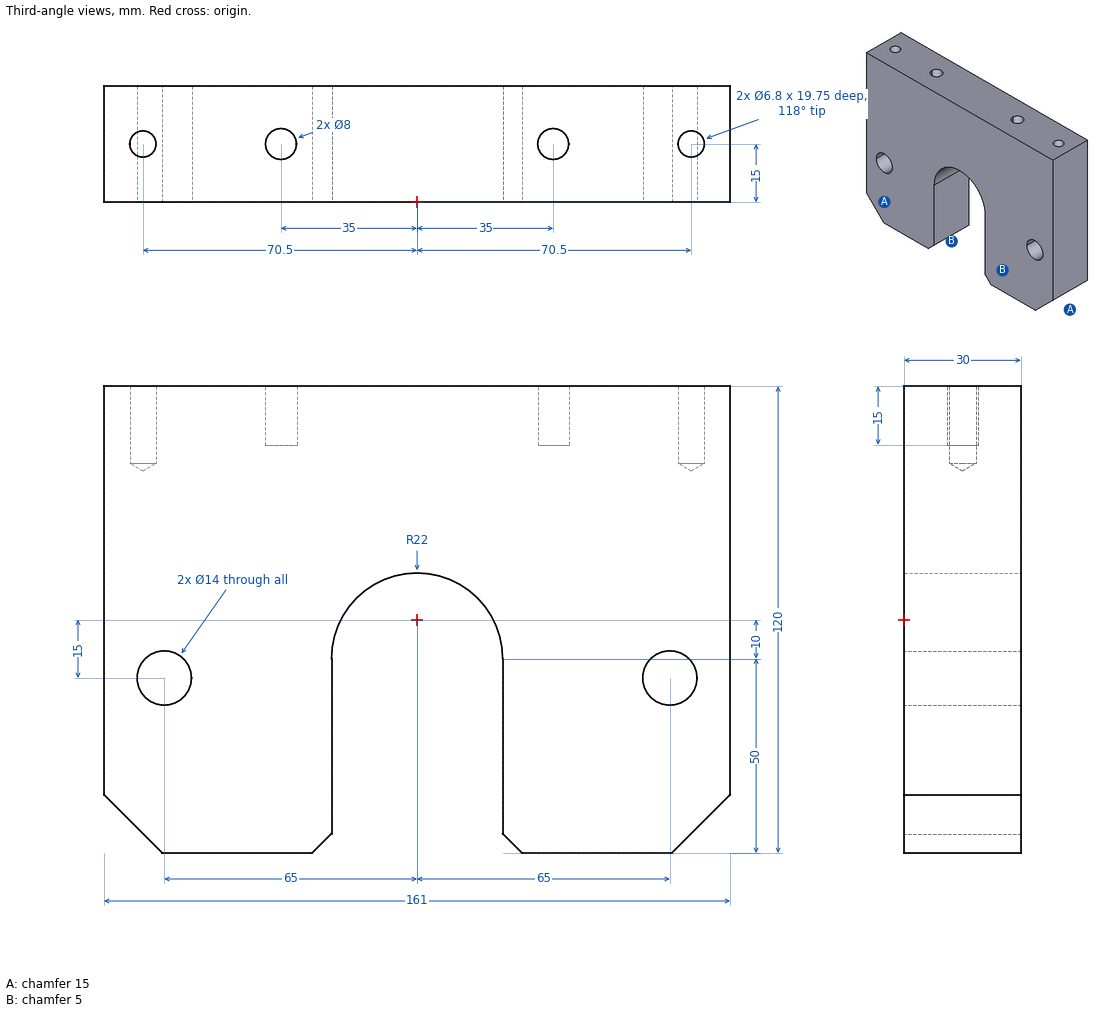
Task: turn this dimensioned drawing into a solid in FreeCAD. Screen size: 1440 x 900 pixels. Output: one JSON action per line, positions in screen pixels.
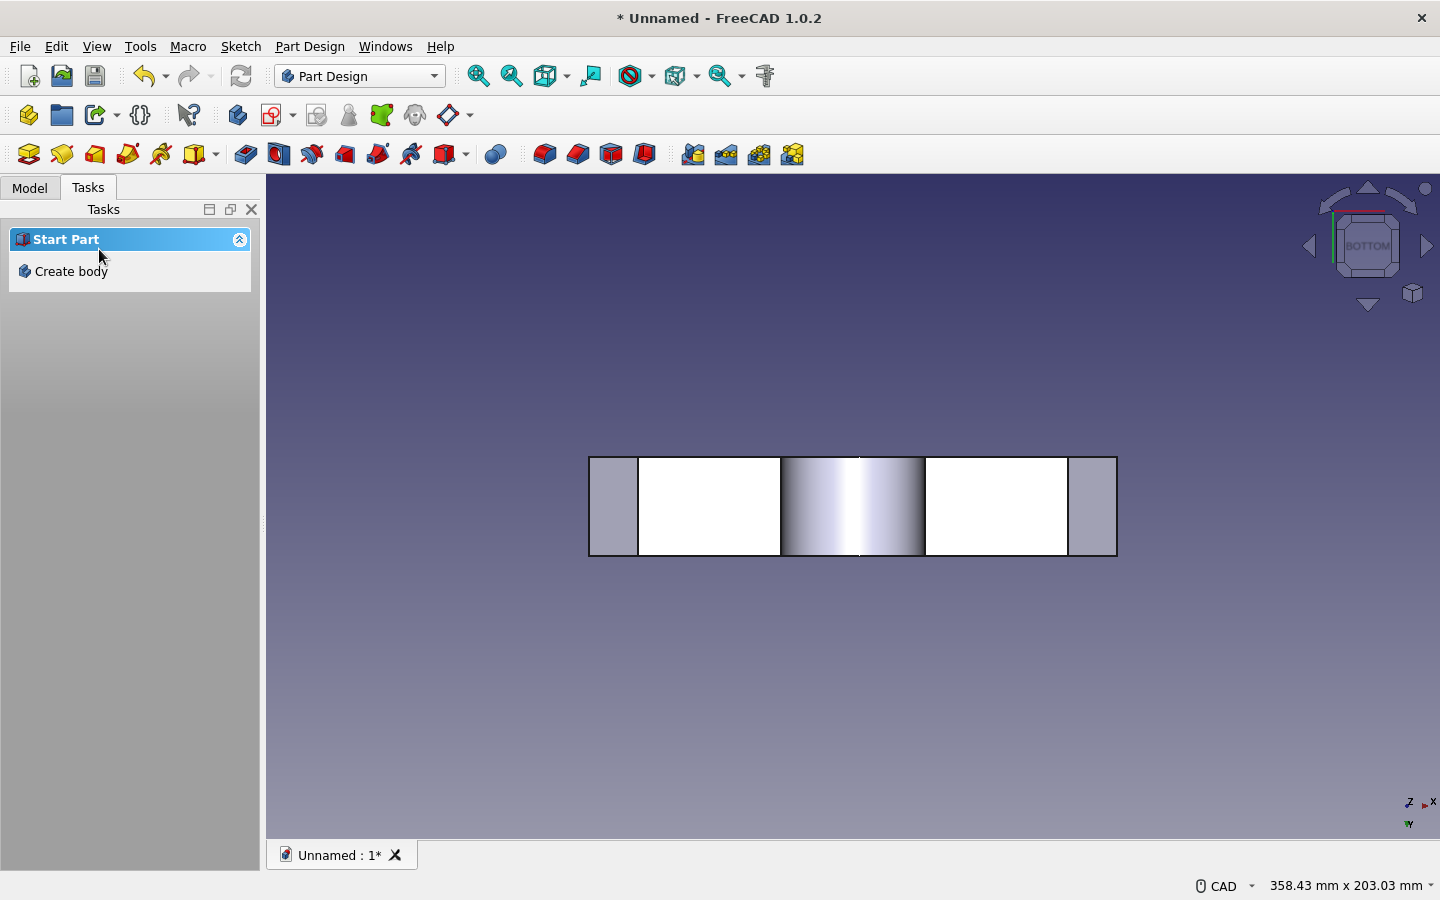
{"action": "key", "text": "v f"}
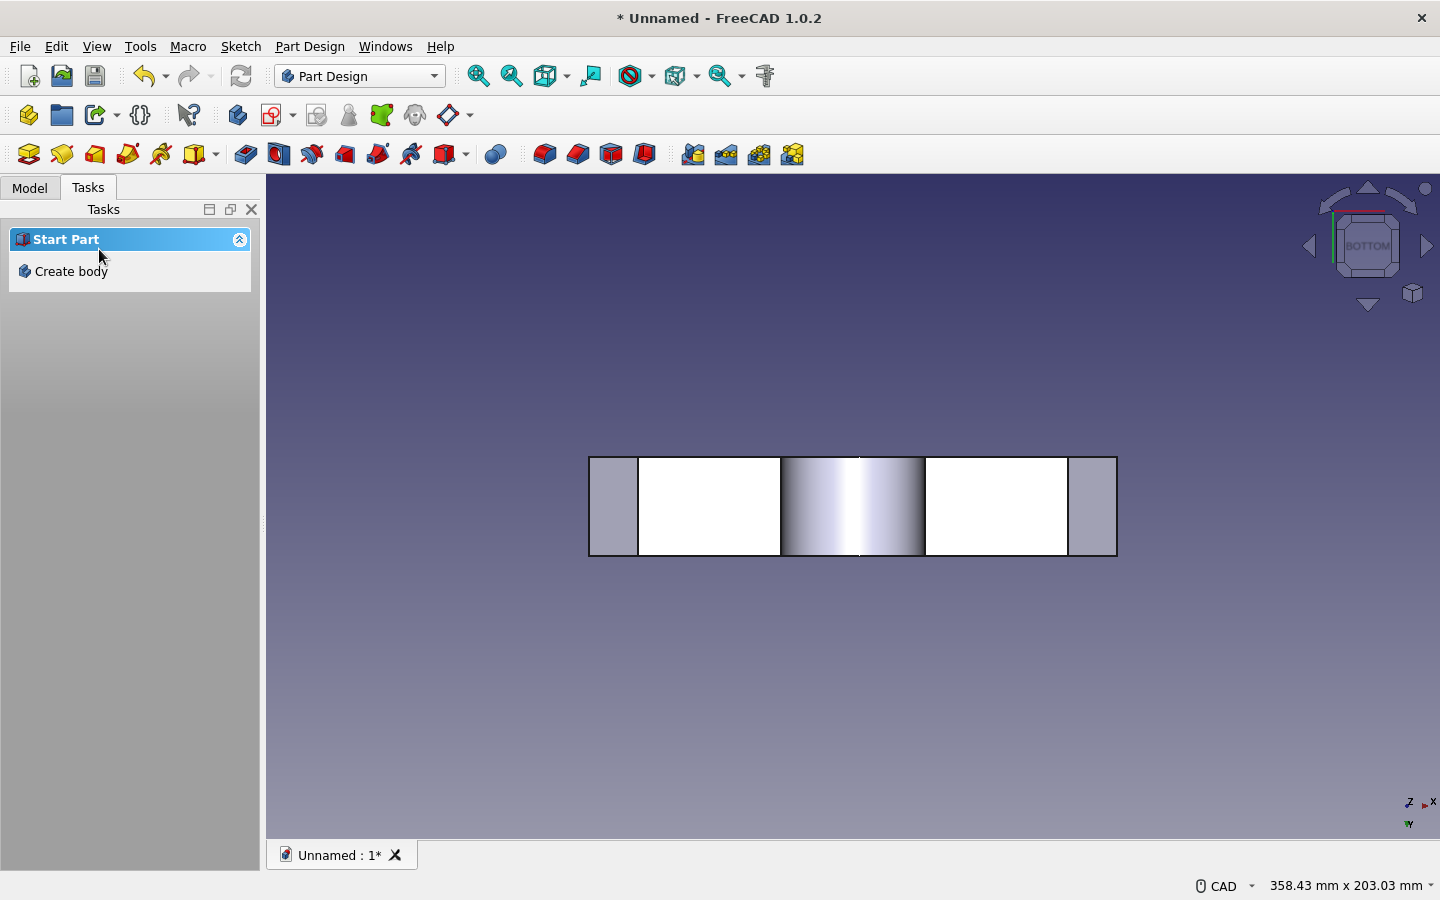
{"action": "left_click", "coordinate": [781, 505]}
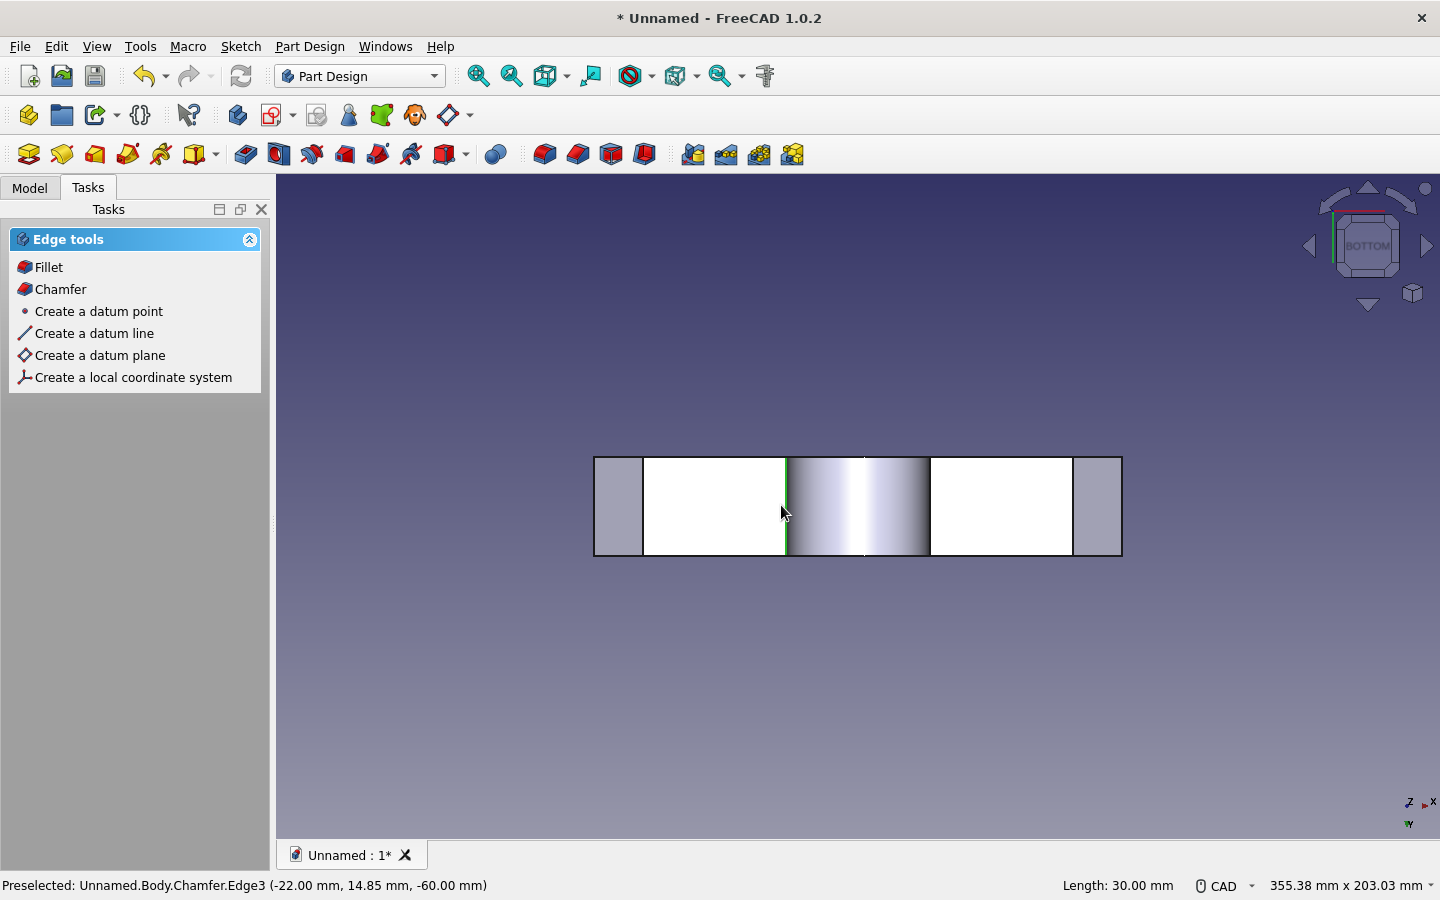
{"action": "left_click", "coordinate": [930, 505], "text": "ctrl"}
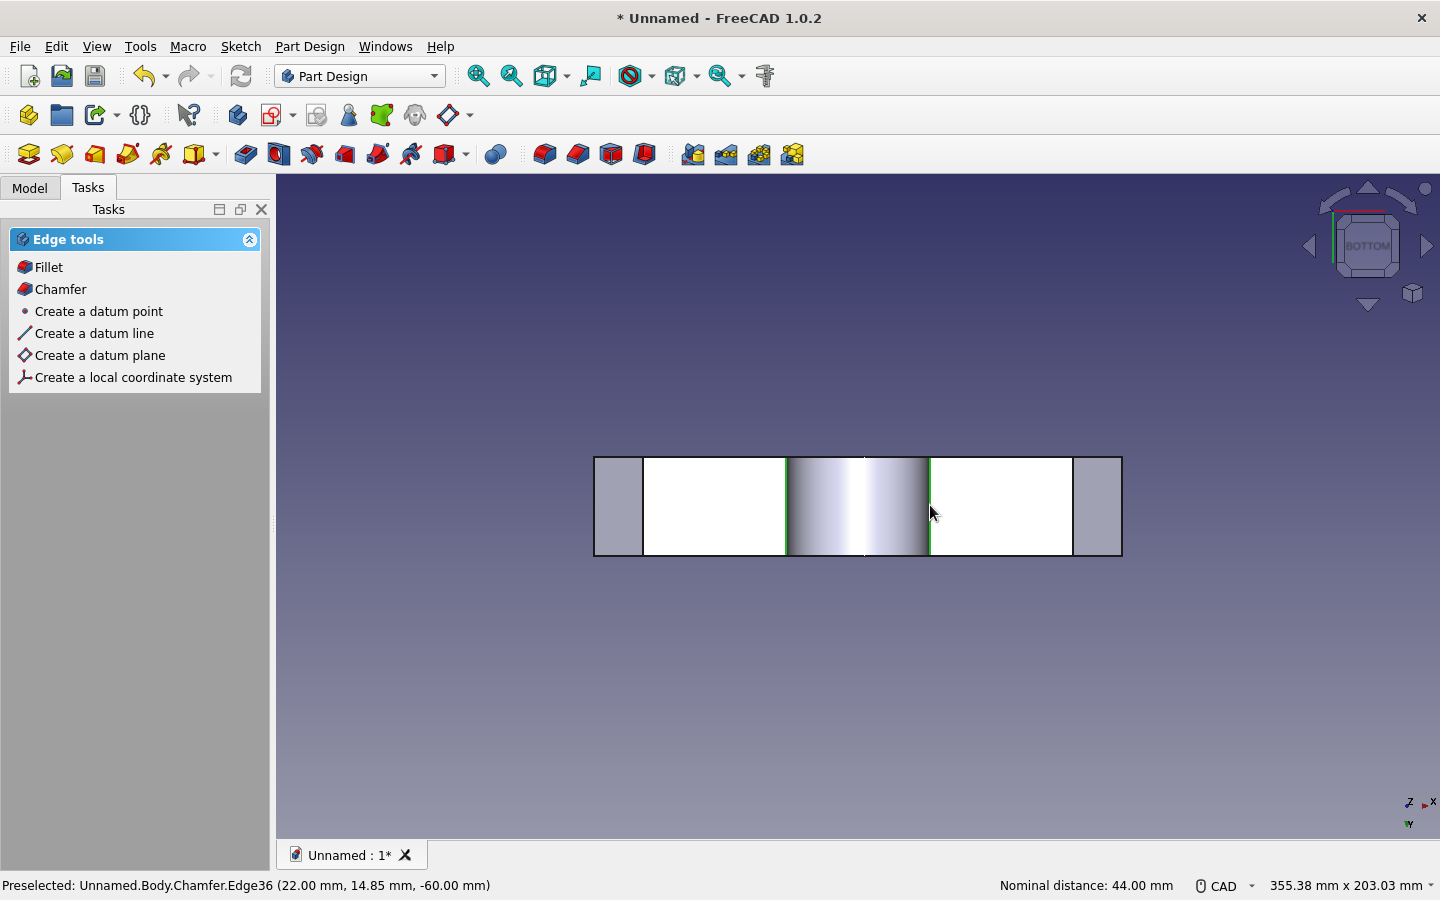
{"action": "left_click", "coordinate": [578, 154]}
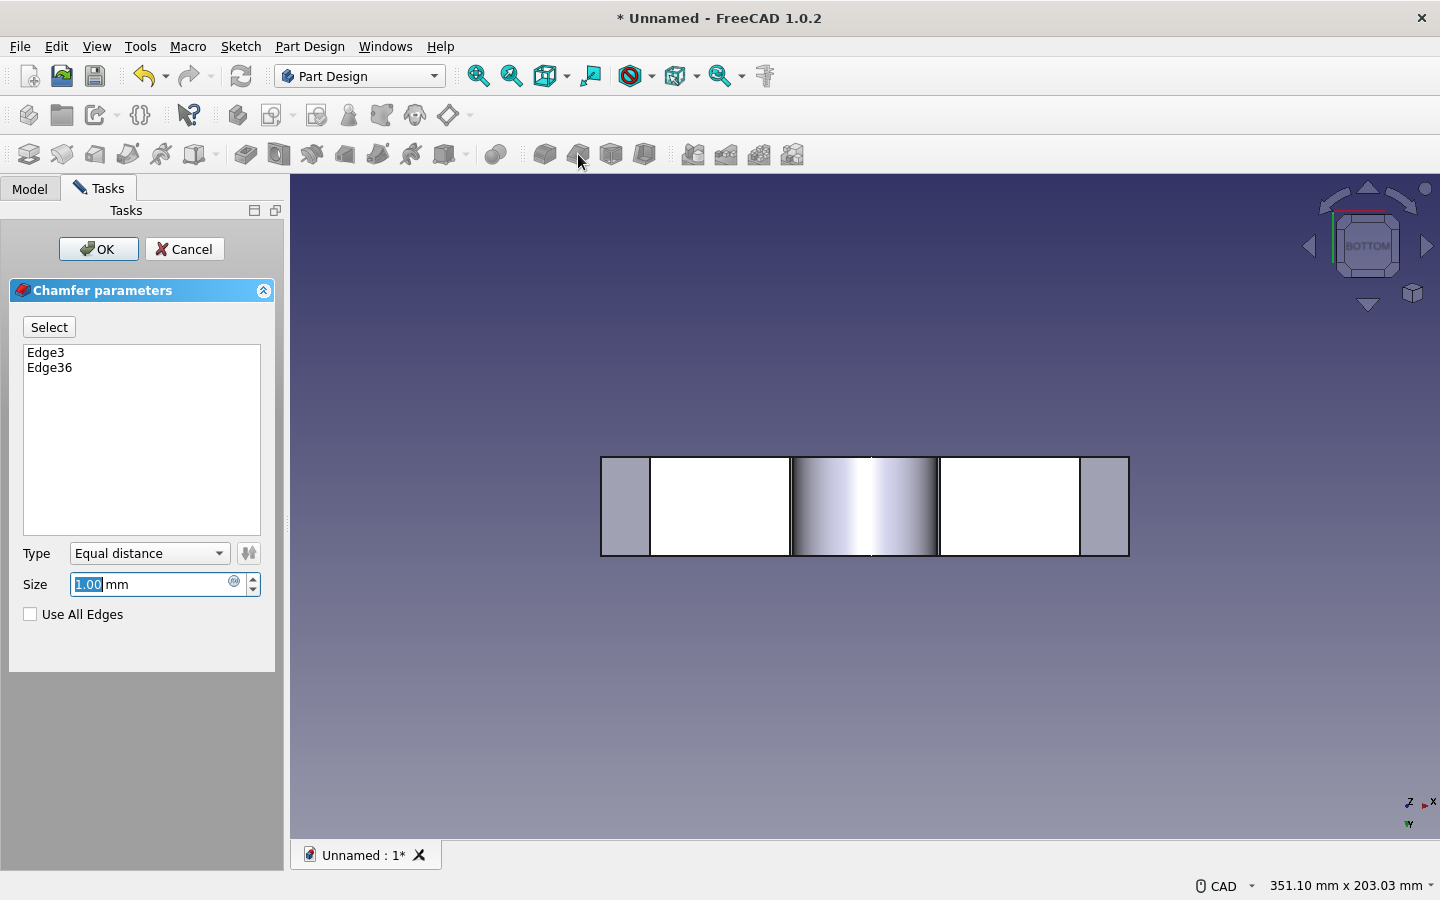
{"action": "type", "text": "5"}
{"action": "key", "text": "Tab"}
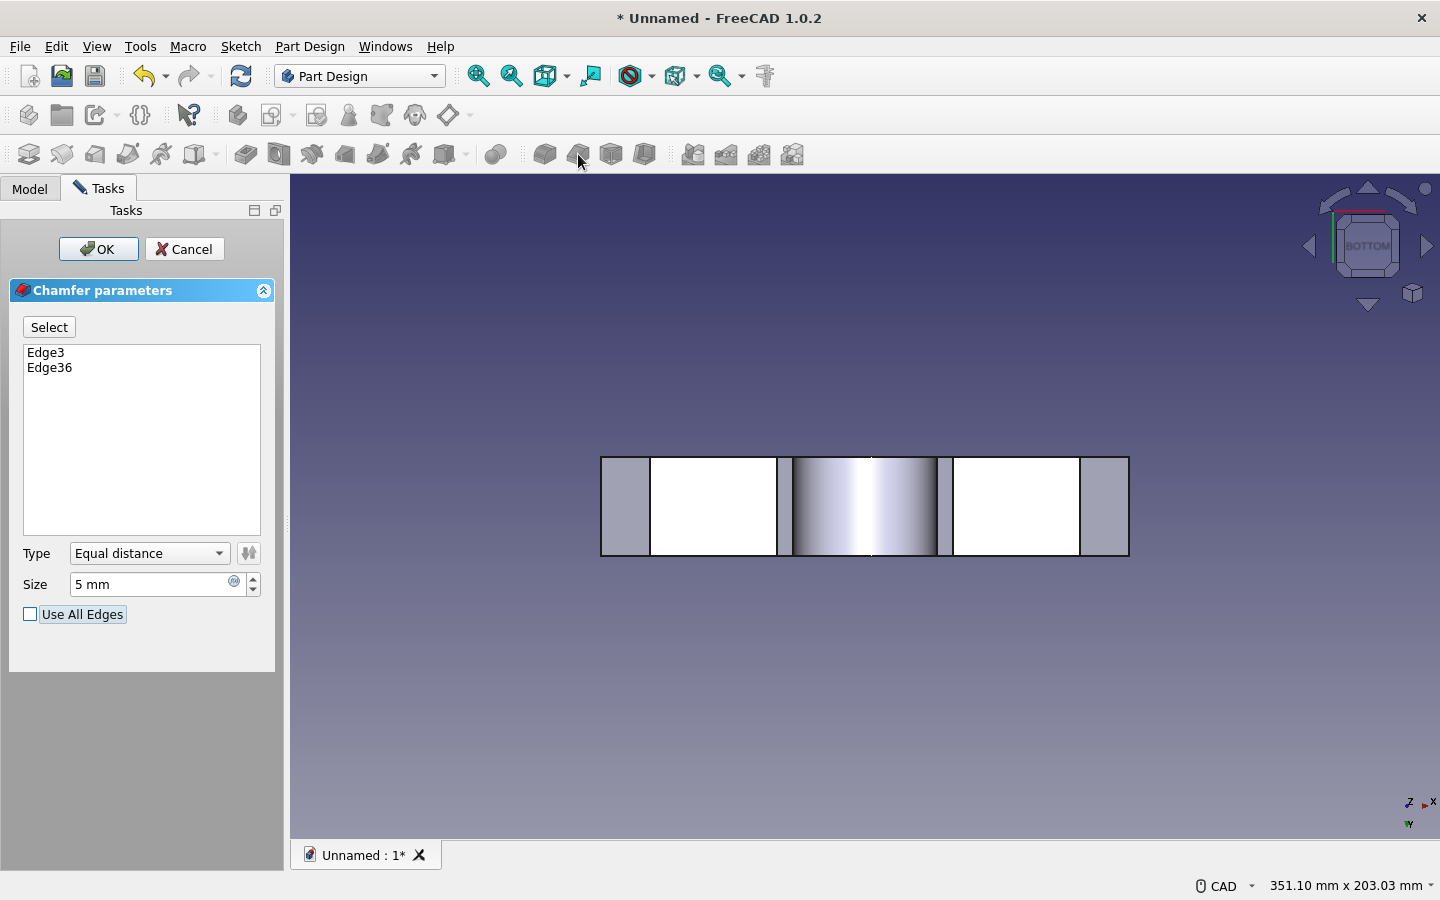
{"action": "left_click", "coordinate": [99, 249]}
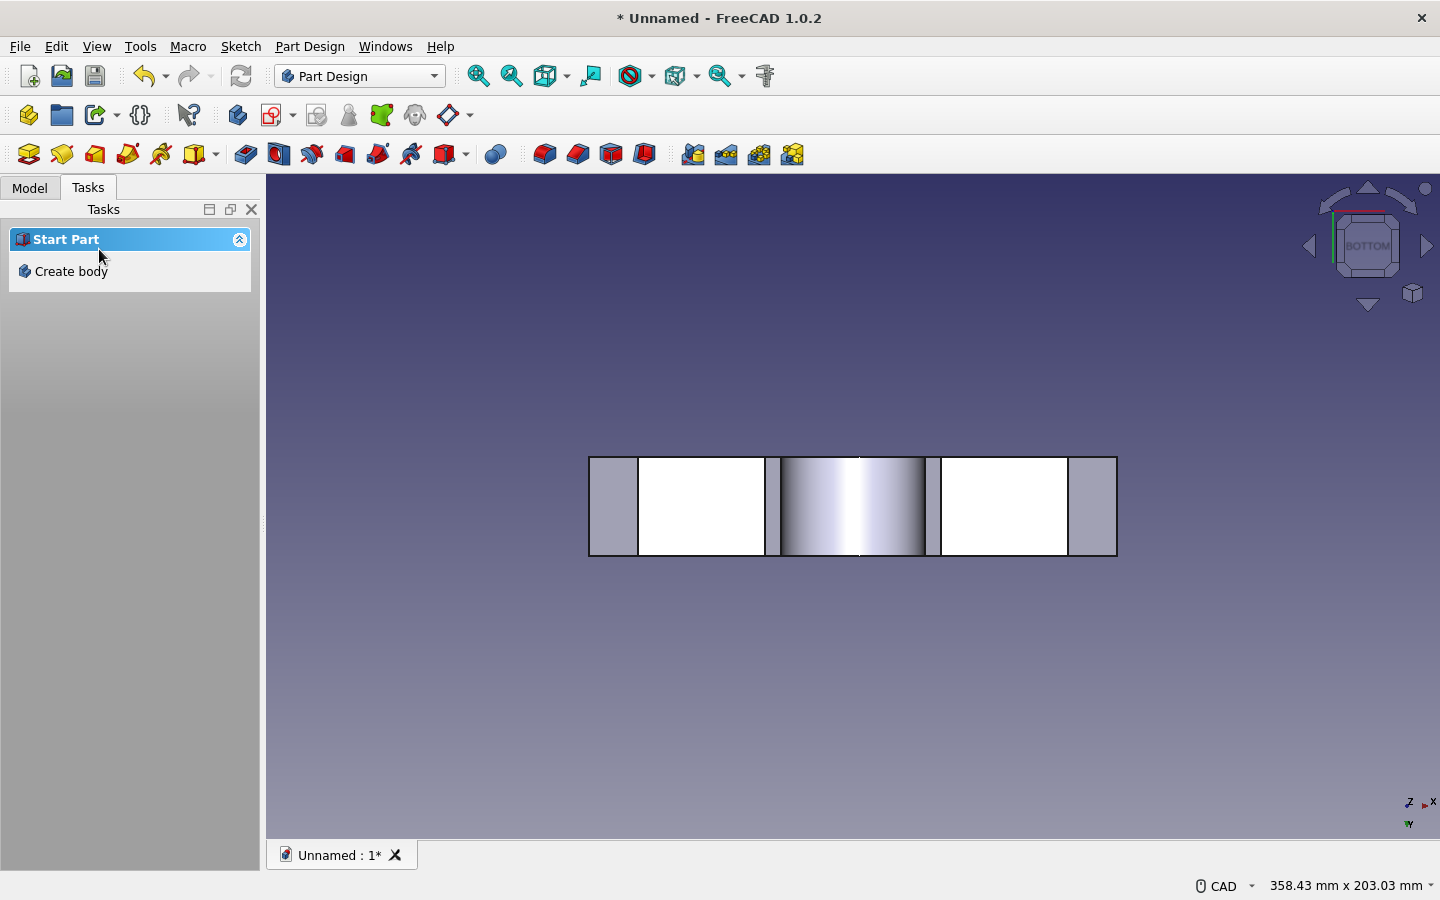
{"action": "key", "text": "0"}